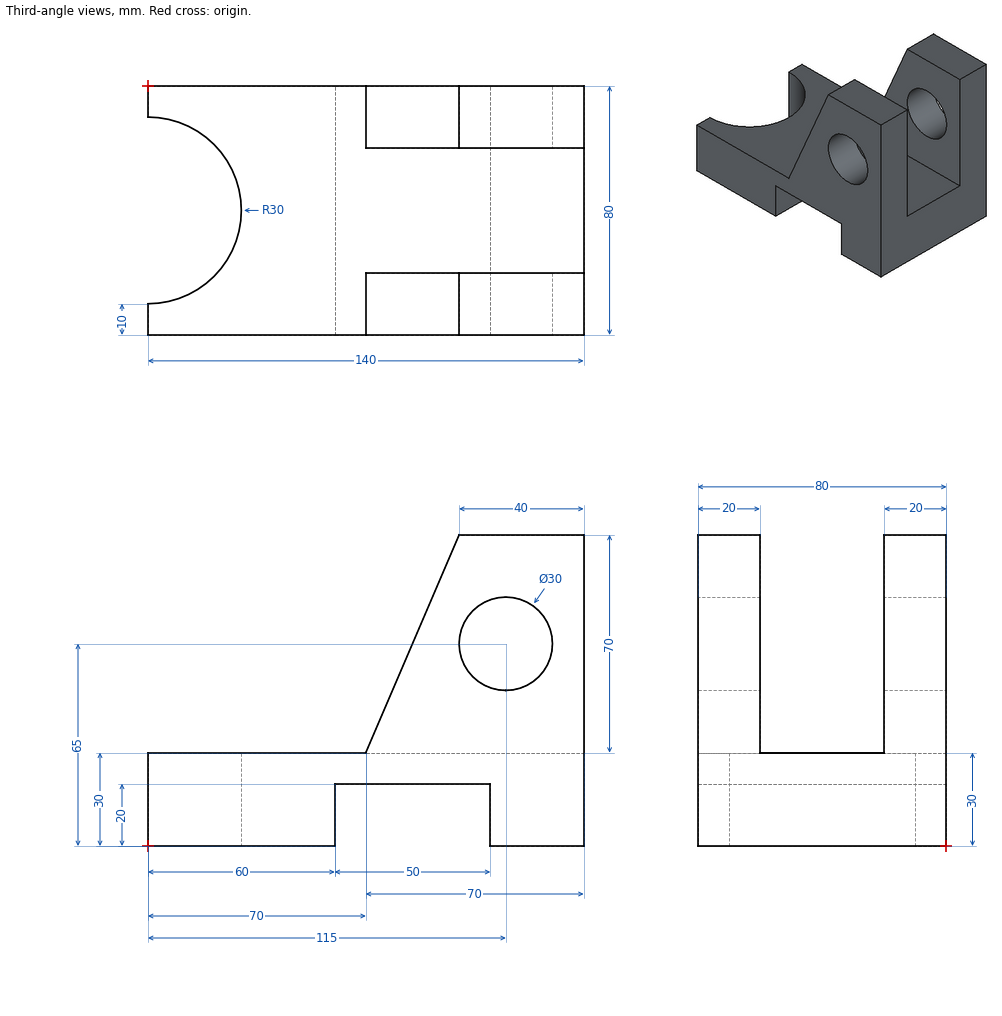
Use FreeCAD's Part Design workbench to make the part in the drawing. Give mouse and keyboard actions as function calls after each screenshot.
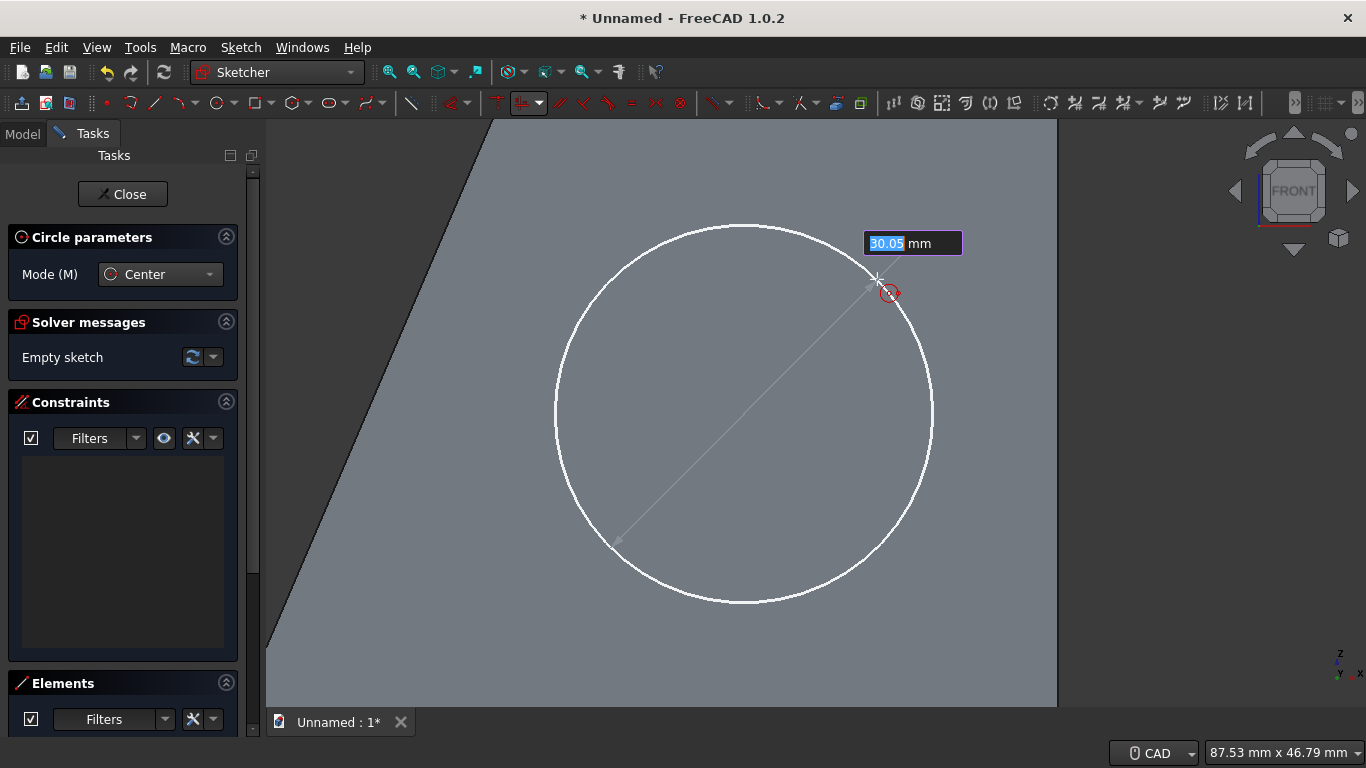
text(30)
key(Return)
key(Escape)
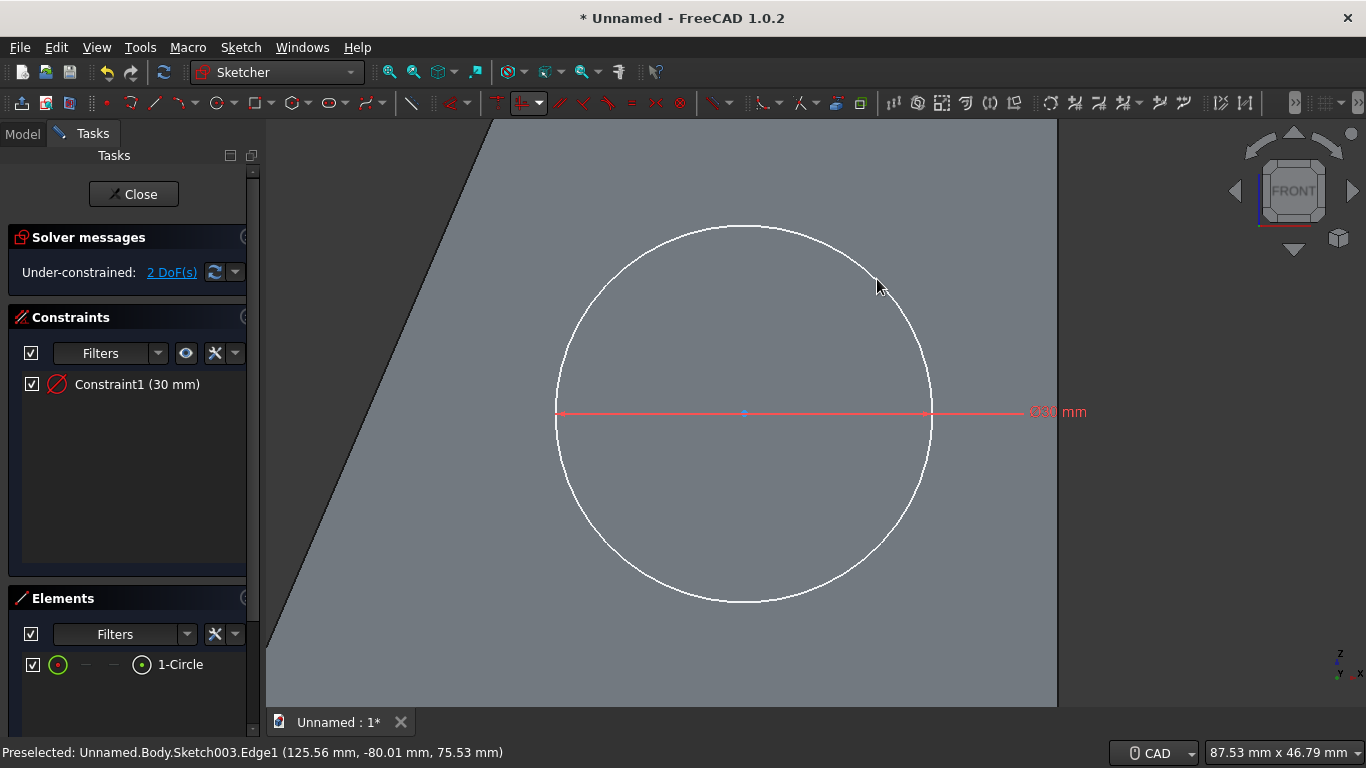
click(450, 104)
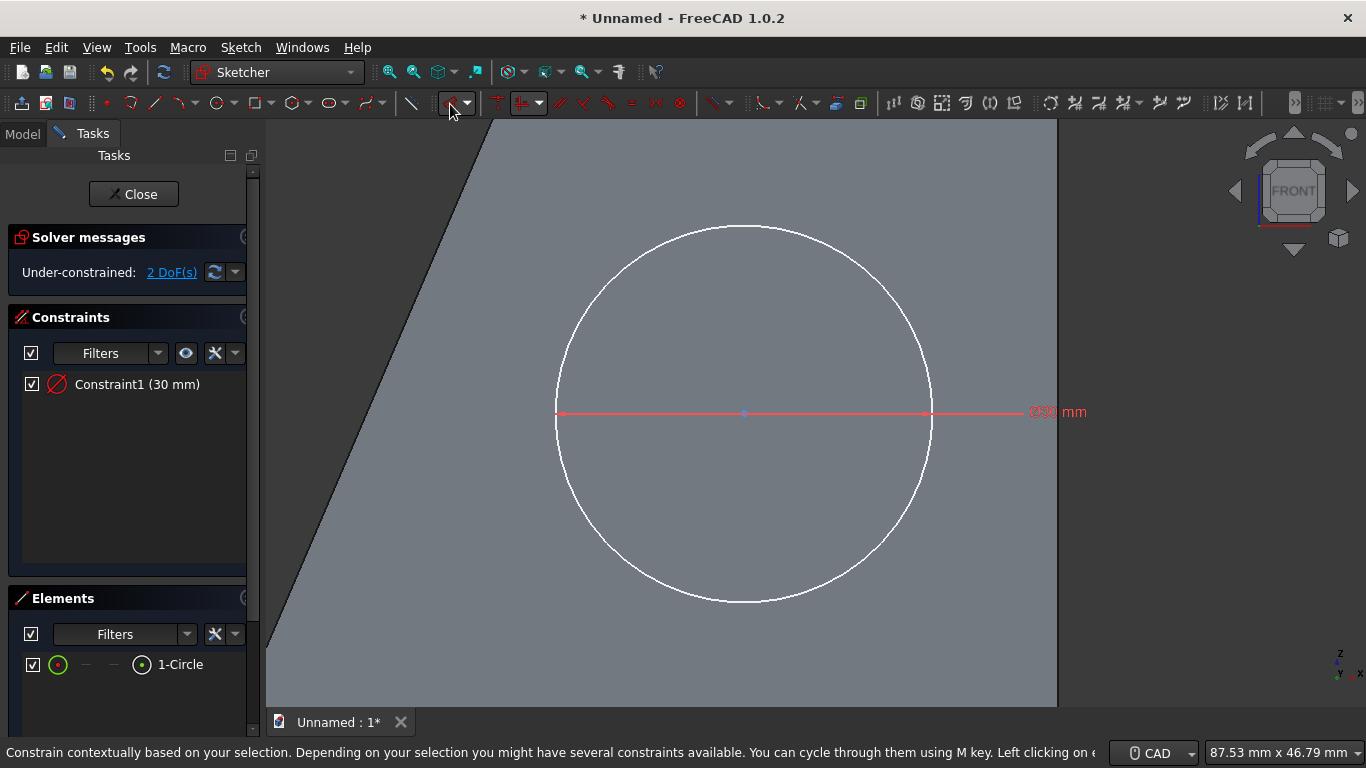
click(744, 414)
click(778, 547)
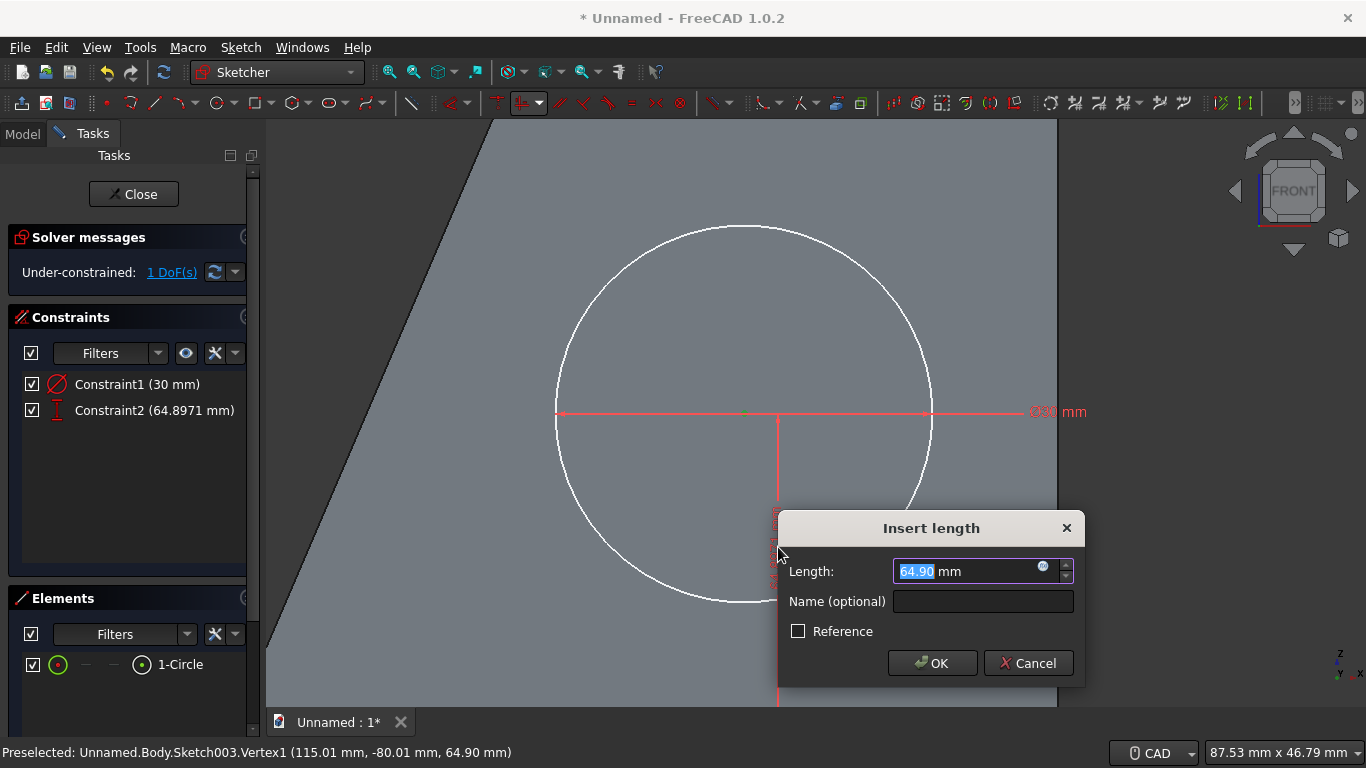
text(65)
key(Return)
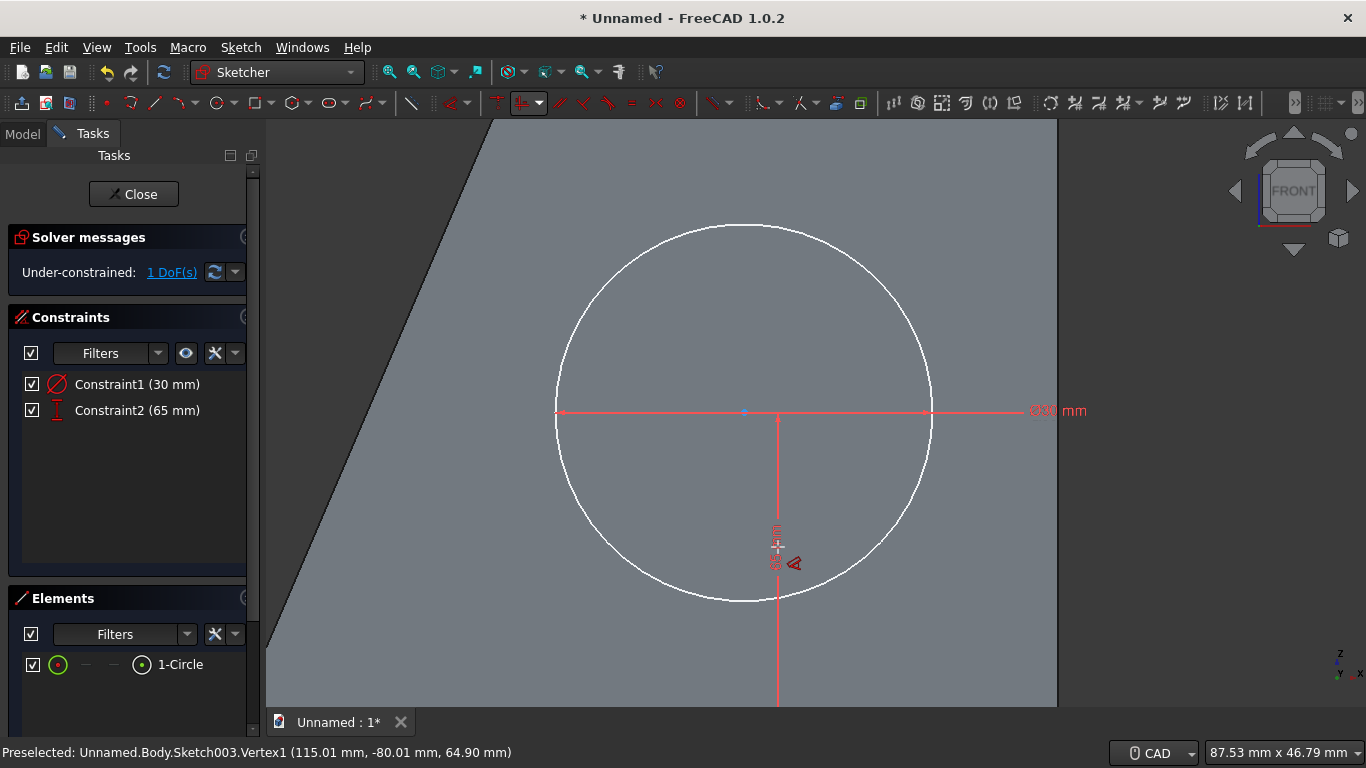
click(744, 413)
click(519, 379)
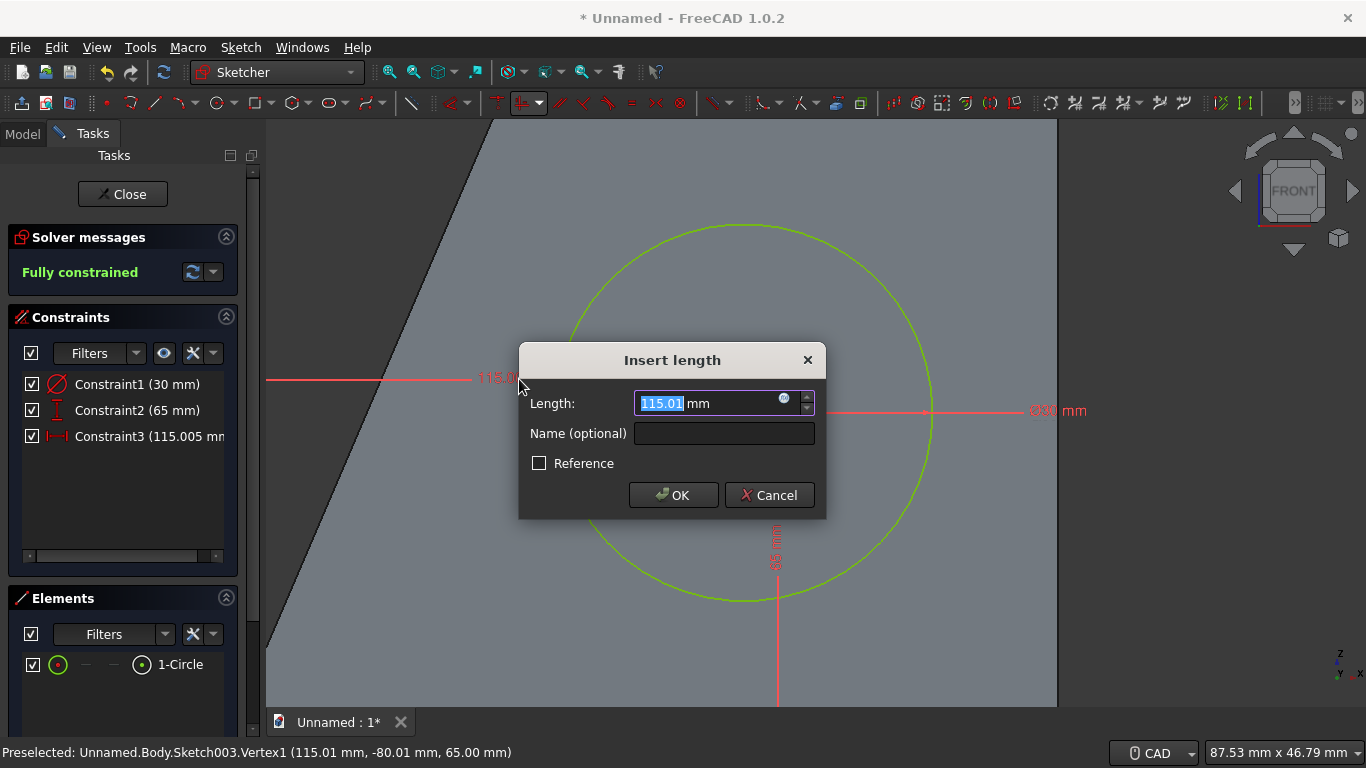
text(115)
key(Return)
key(Escape)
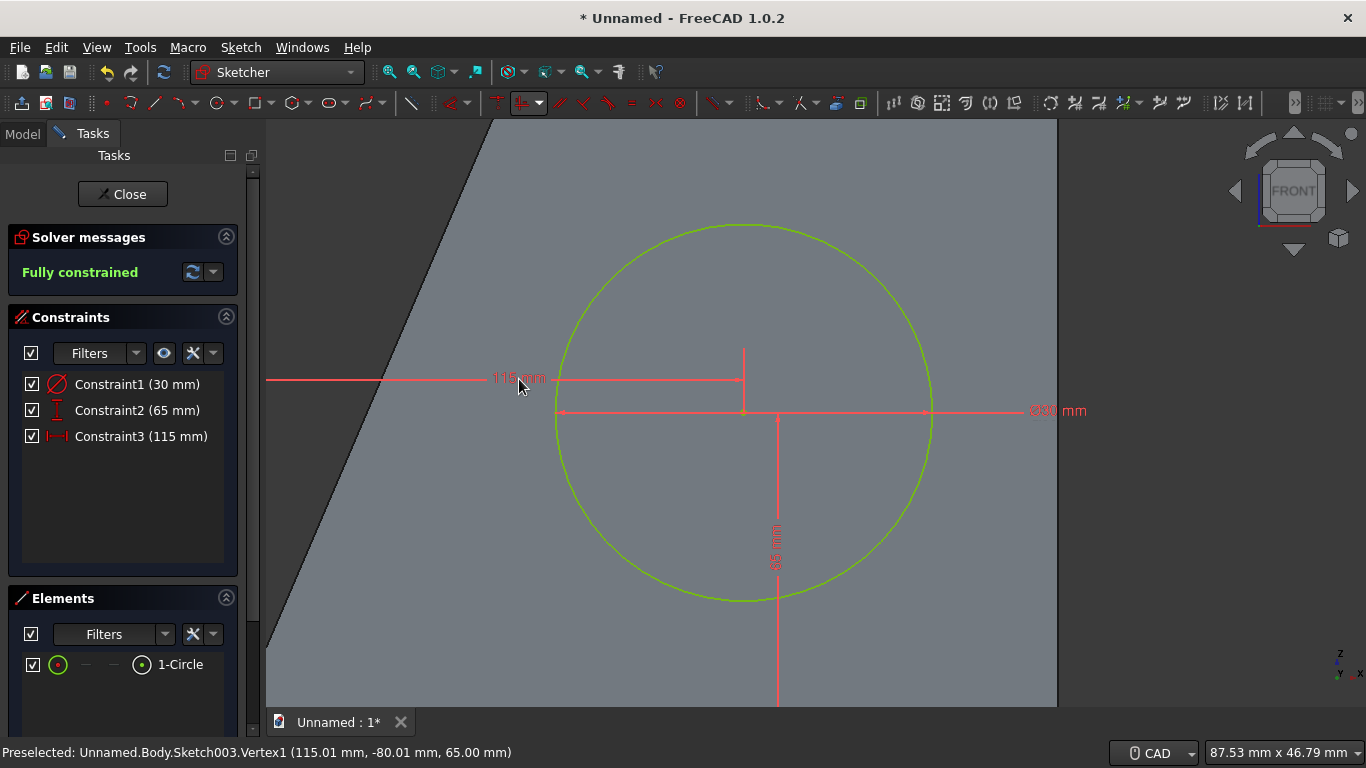
click(123, 194)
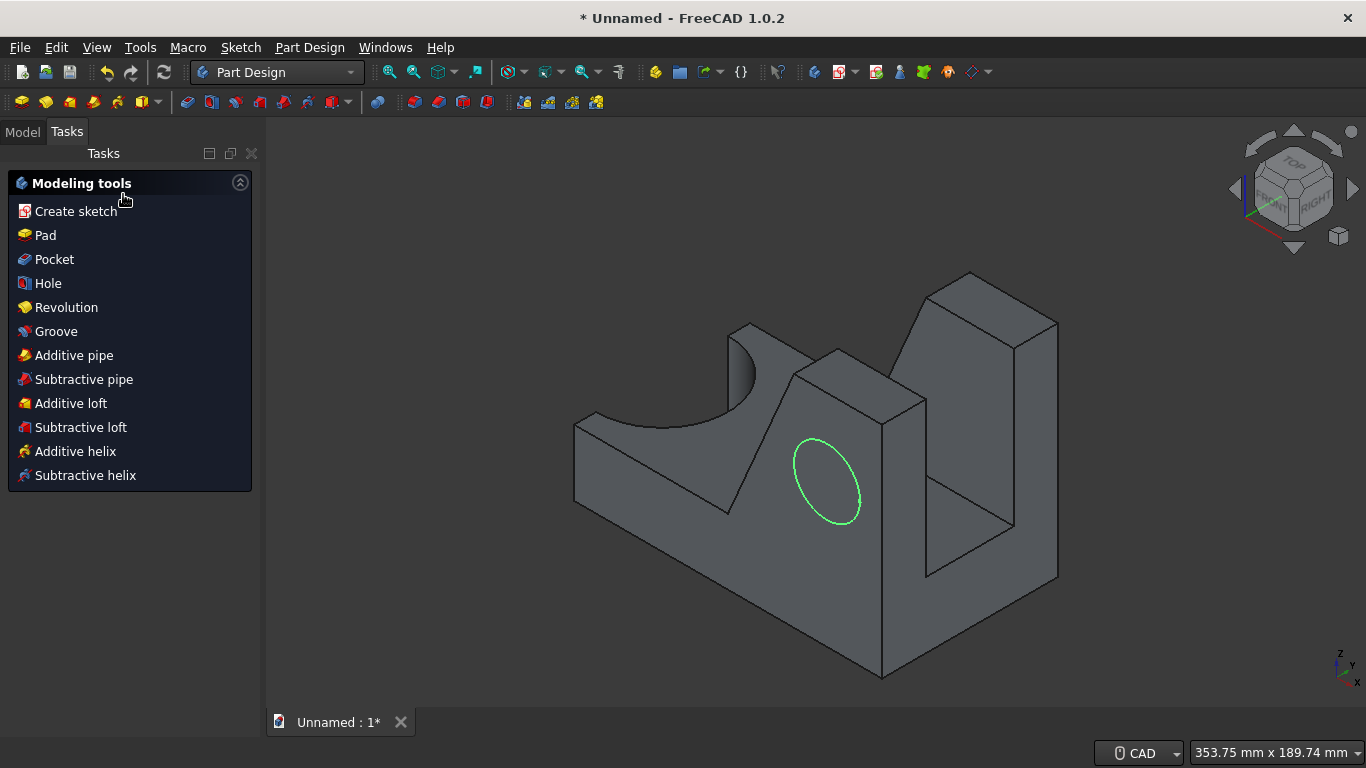
click(188, 102)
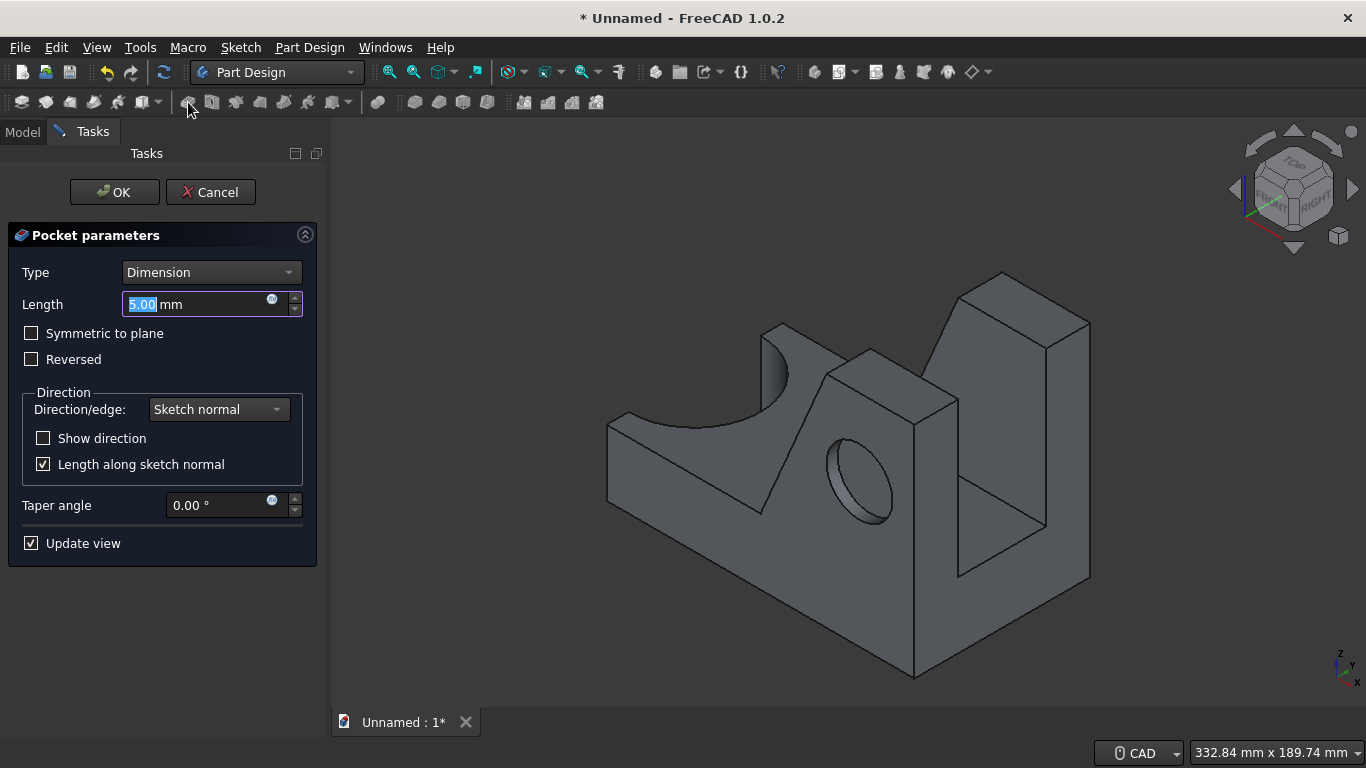
text(80)
key(Tab)